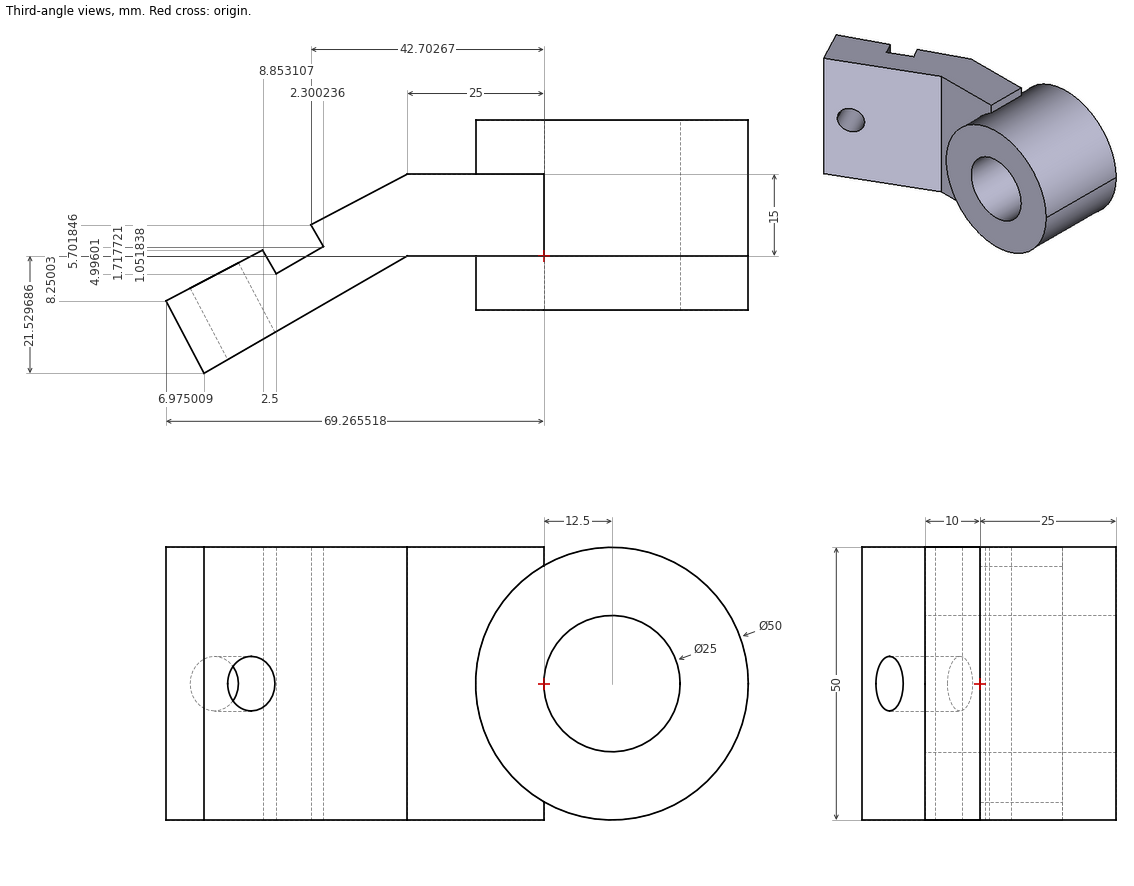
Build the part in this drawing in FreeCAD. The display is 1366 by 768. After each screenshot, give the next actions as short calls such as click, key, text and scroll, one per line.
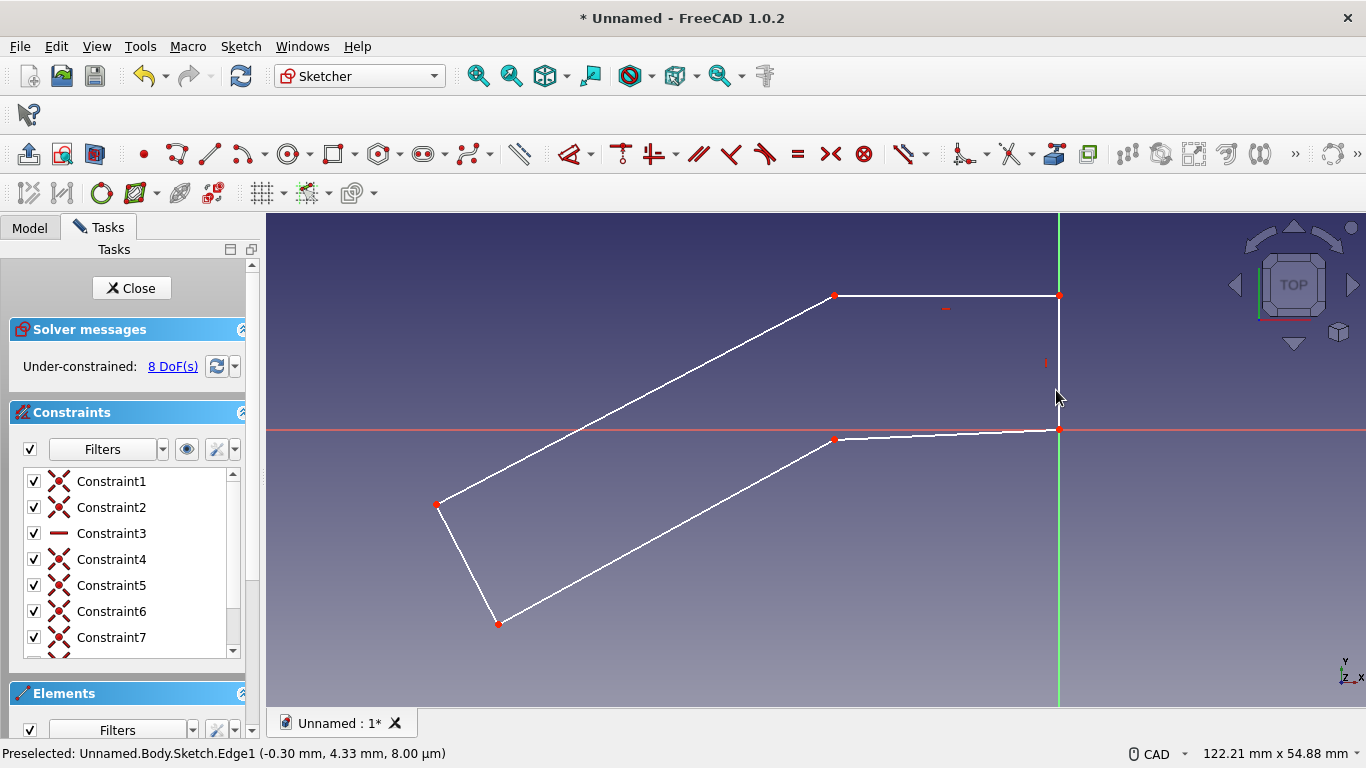
click(992, 433)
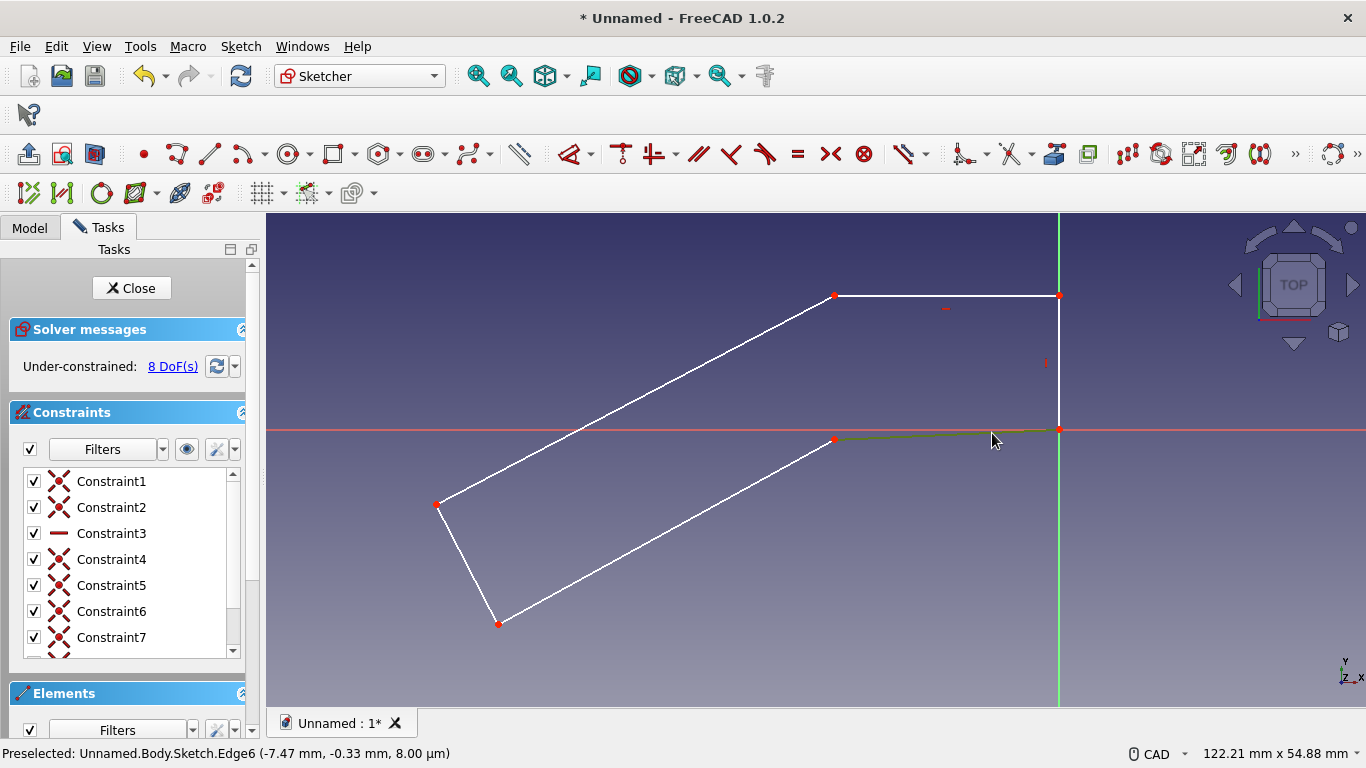
click(676, 154)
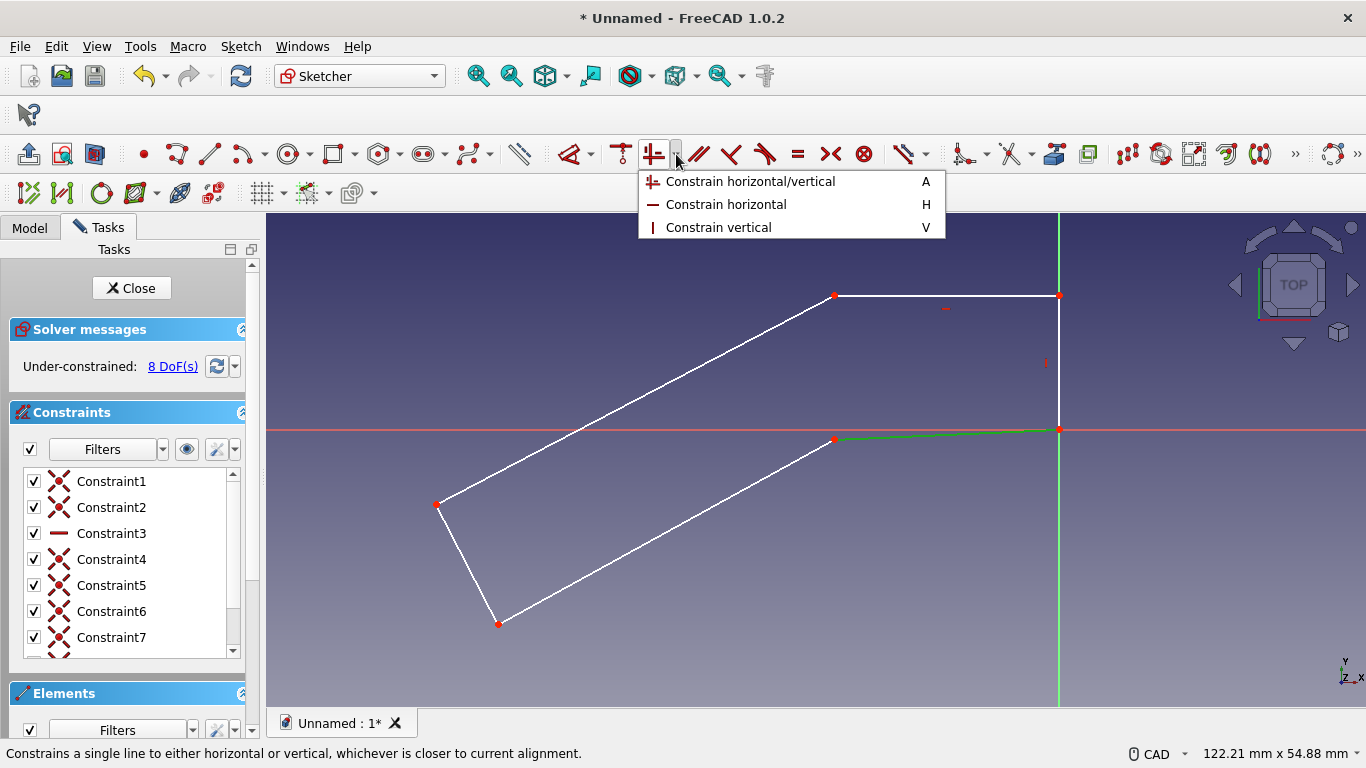
click(792, 204)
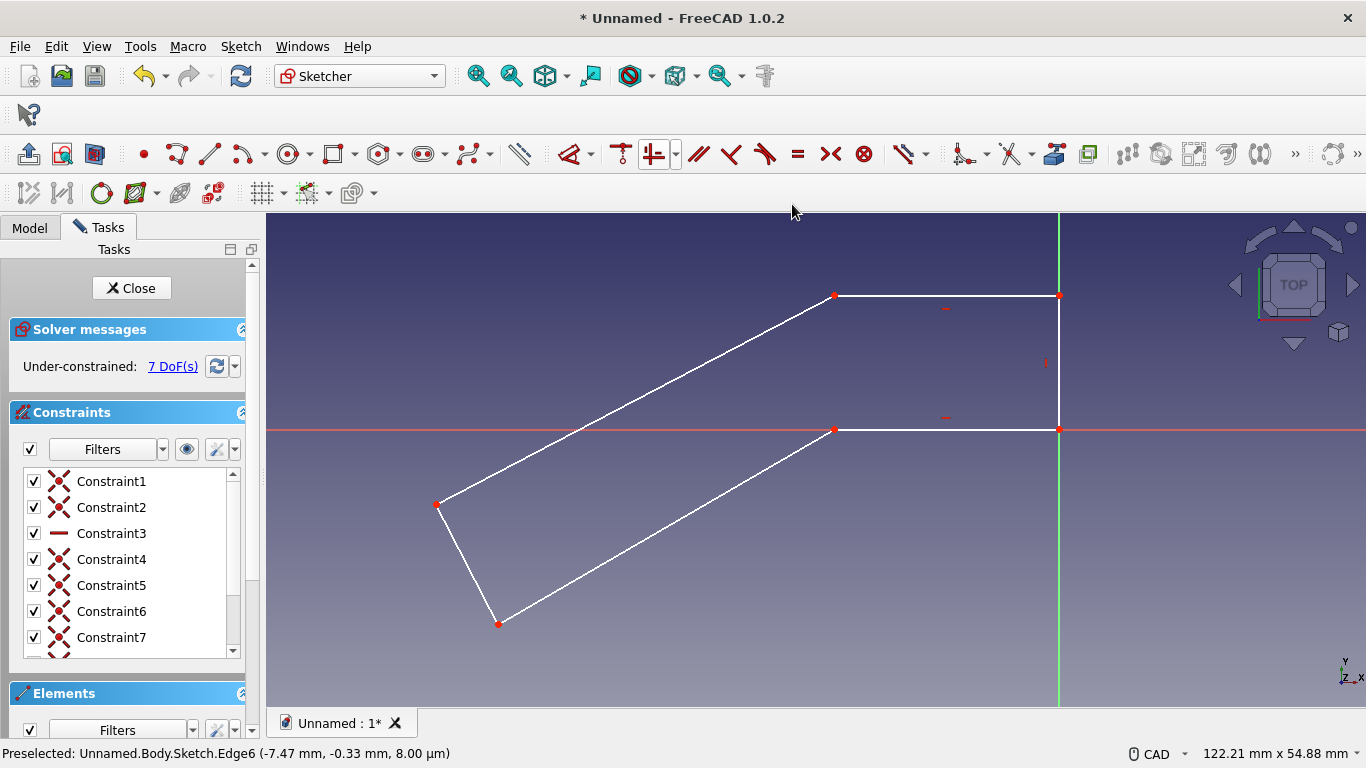
click(568, 154)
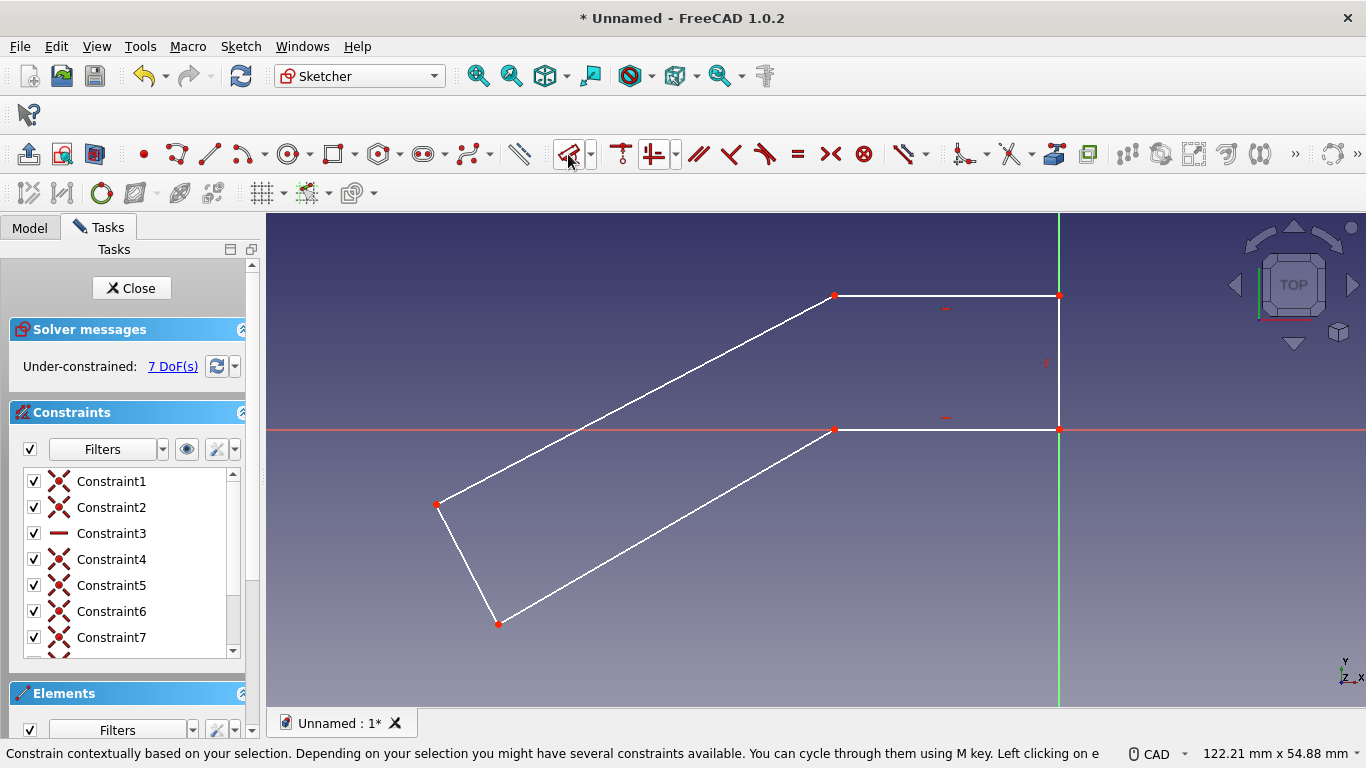
click(1059, 390)
click(1093, 363)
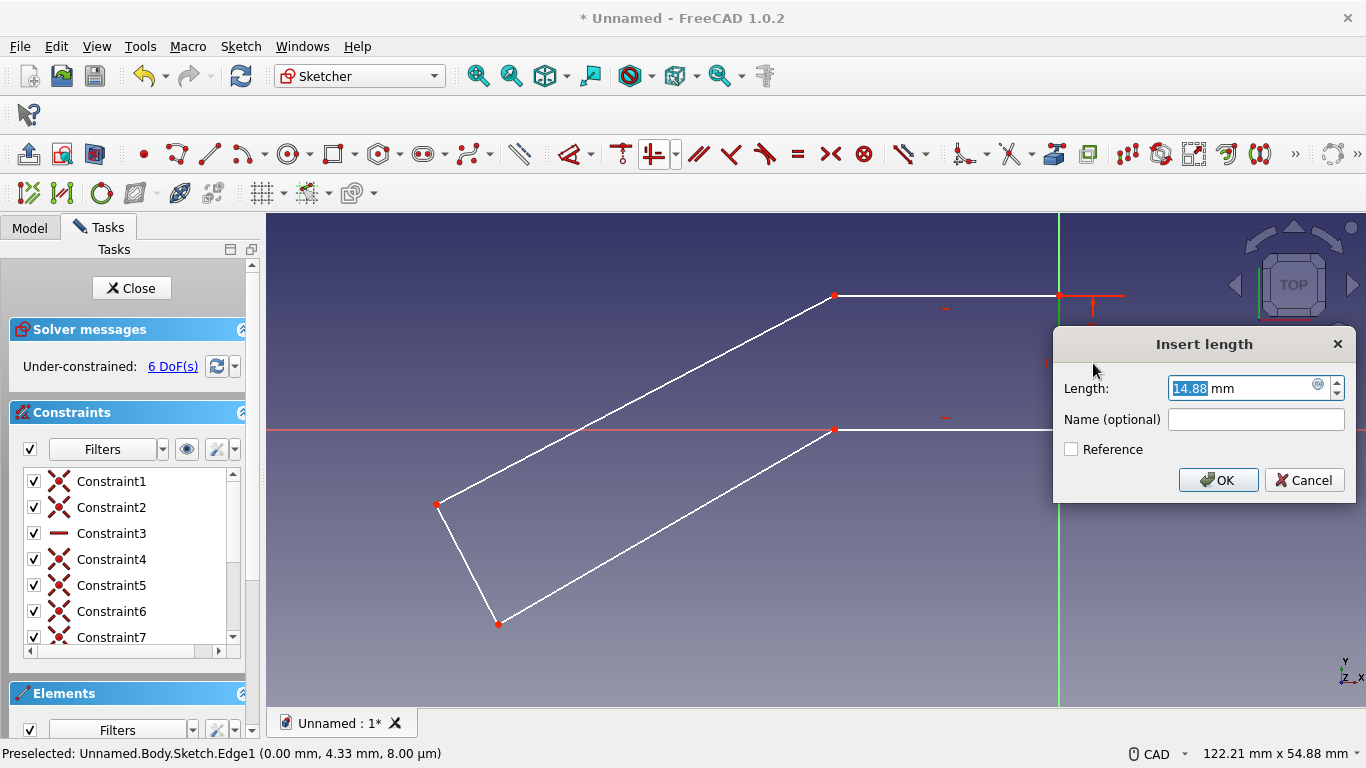
text(15)
key(Return)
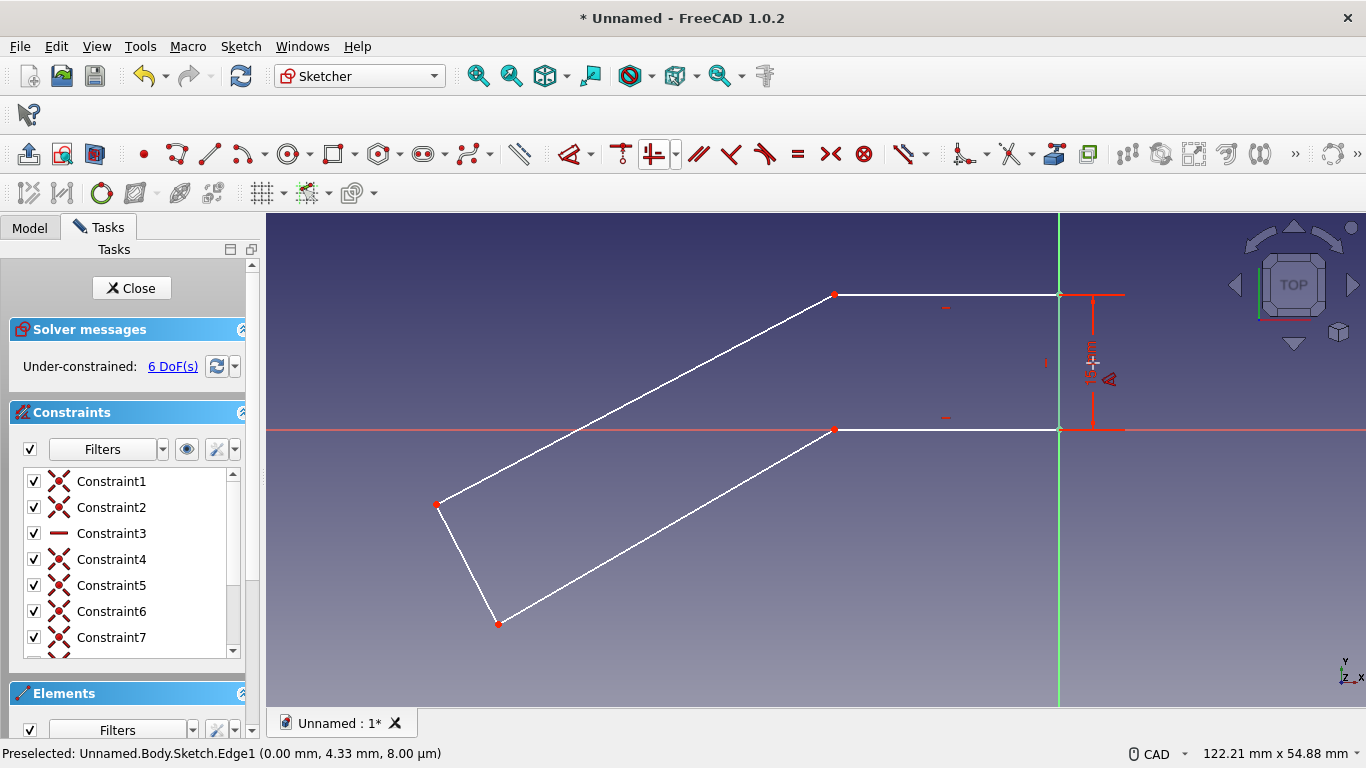
click(992, 295)
click(947, 261)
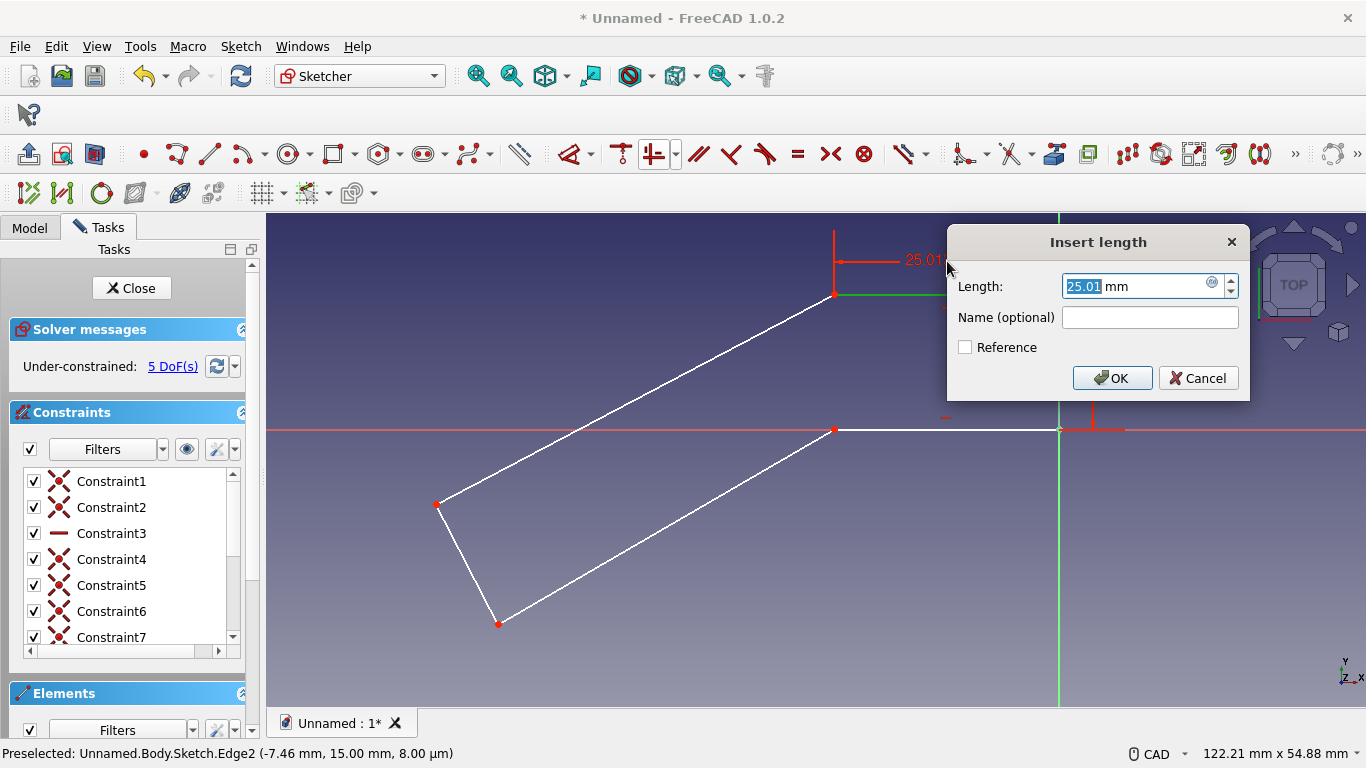
text(25)
key(Return)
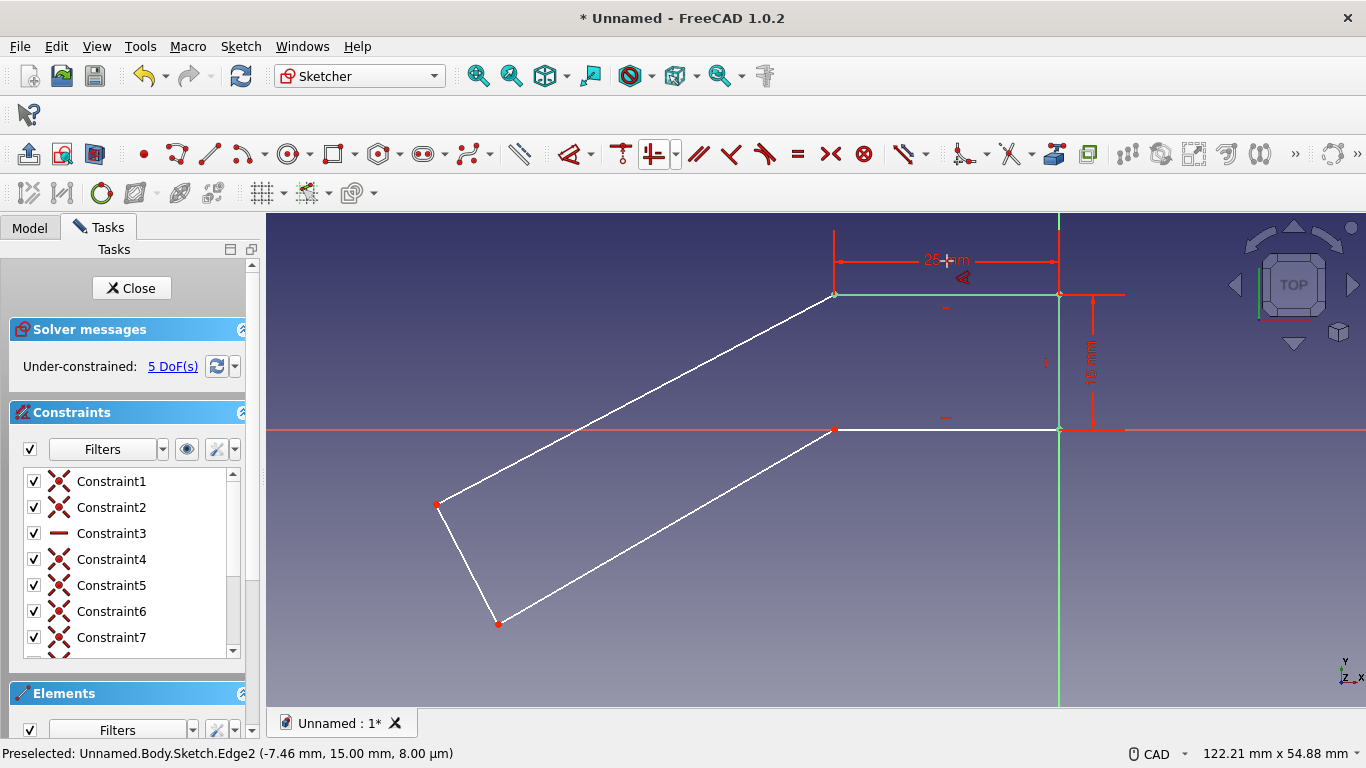
click(902, 430)
click(947, 396)